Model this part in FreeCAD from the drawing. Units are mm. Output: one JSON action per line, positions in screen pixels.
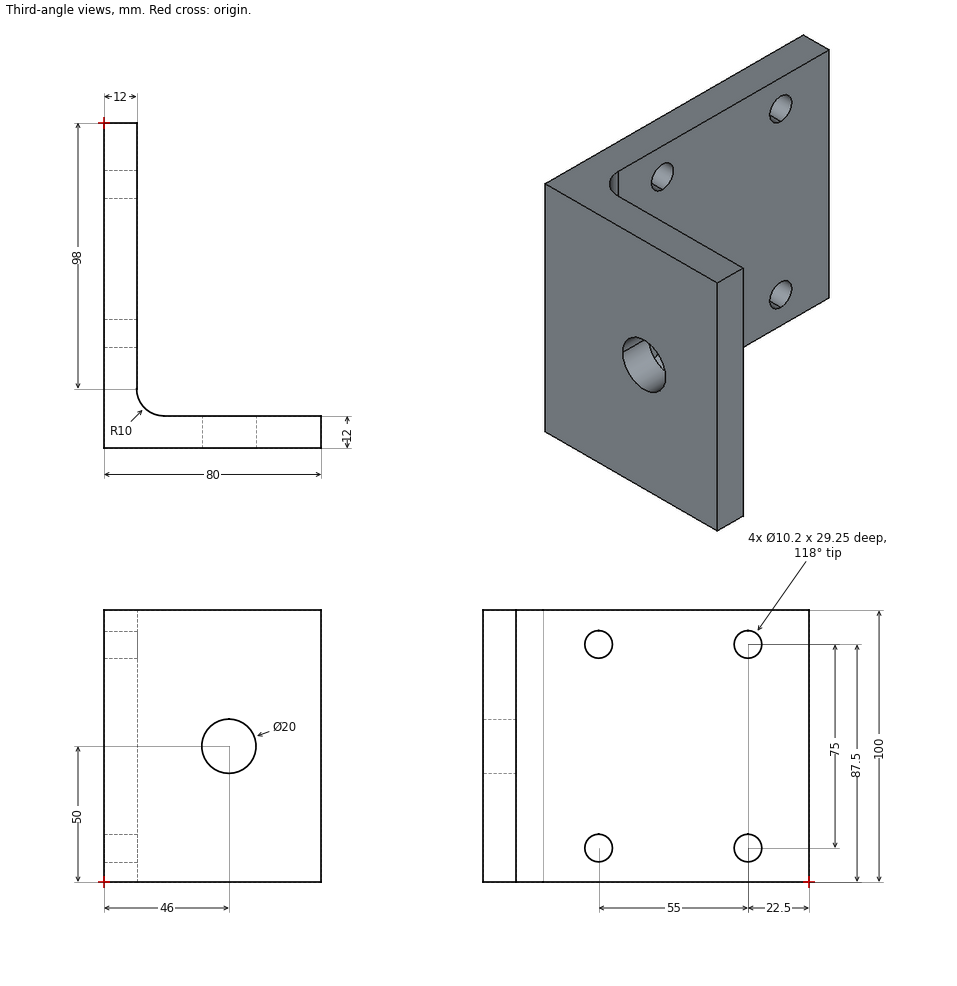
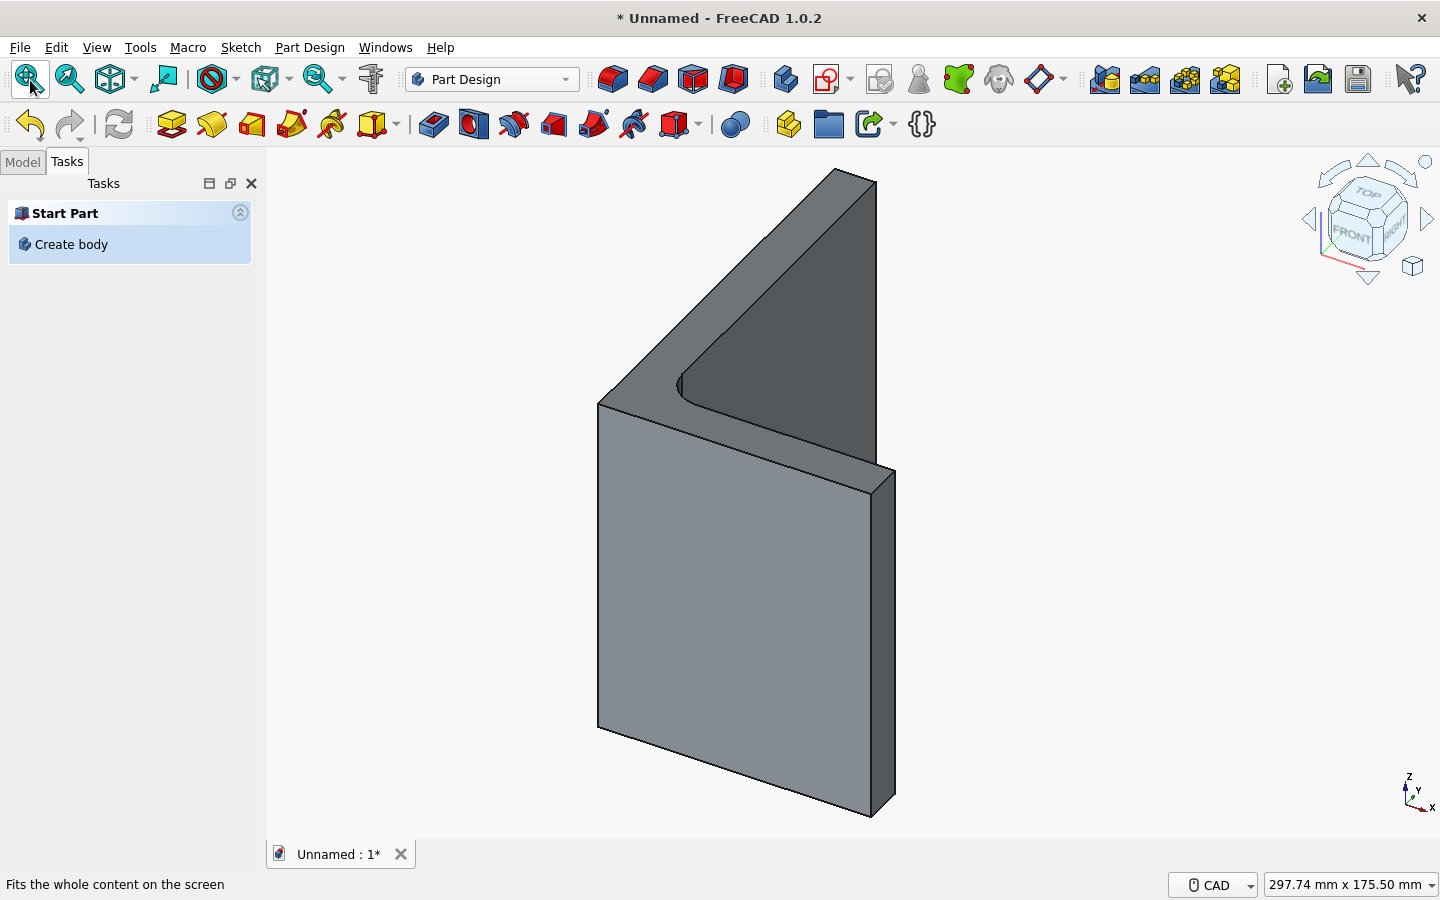
{"action": "left_click", "coordinate": [779, 393]}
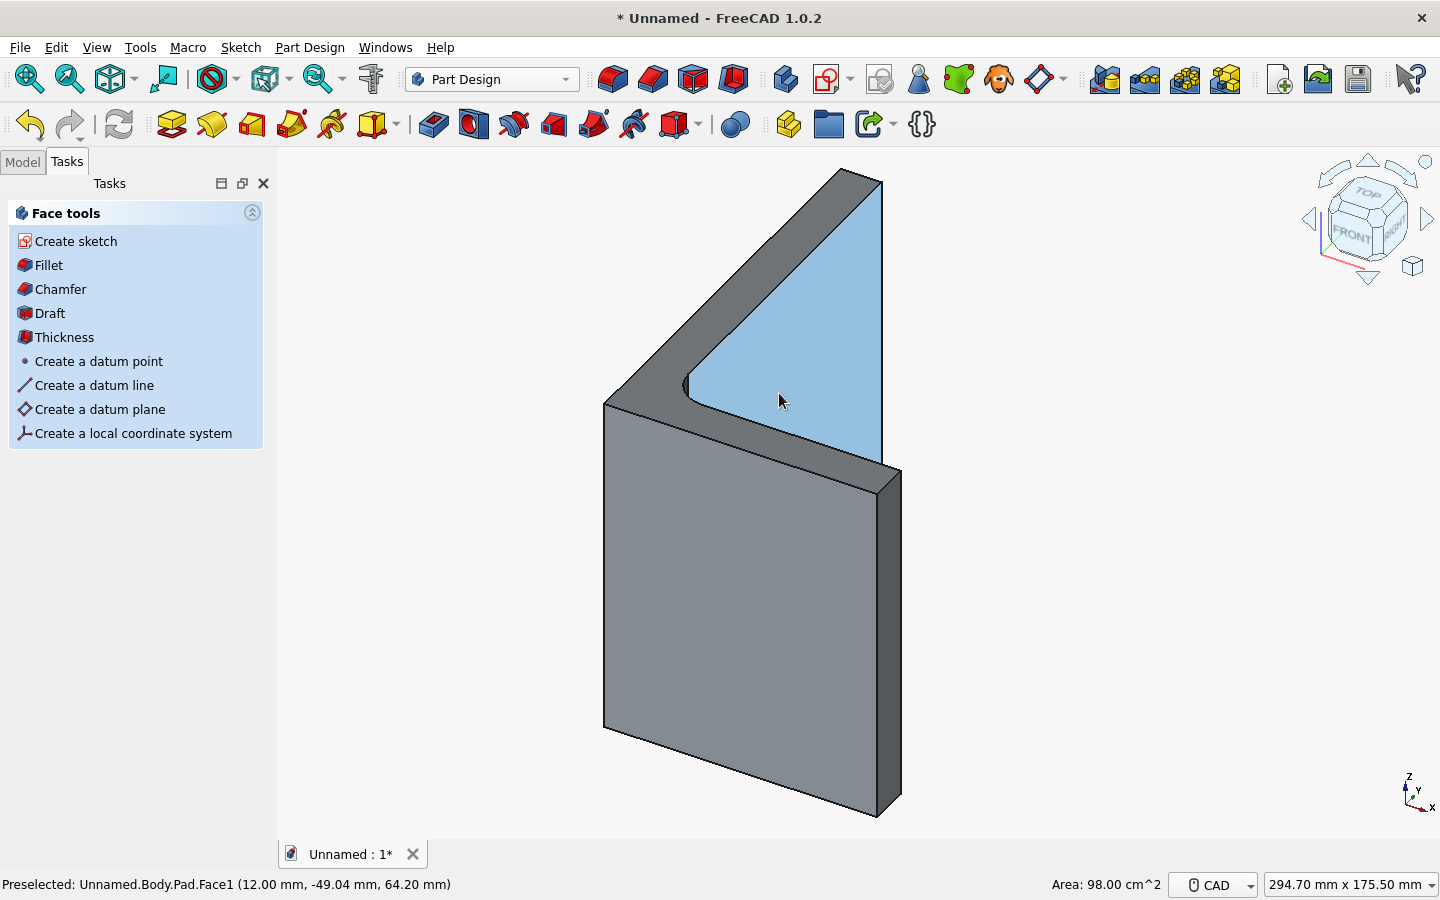
{"action": "left_click", "coordinate": [826, 80]}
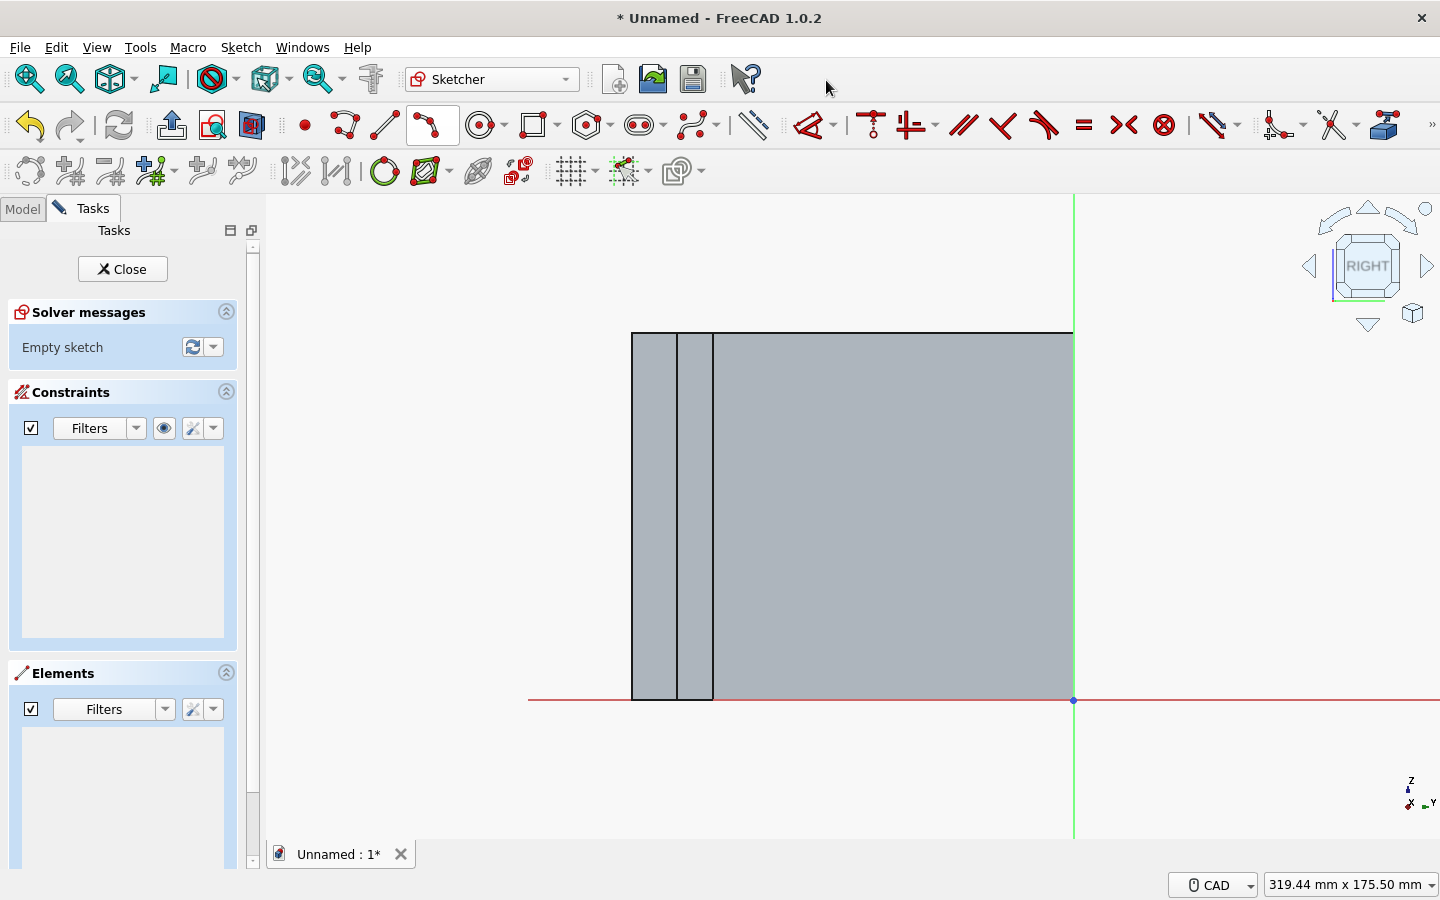
{"action": "left_click", "coordinate": [252, 126]}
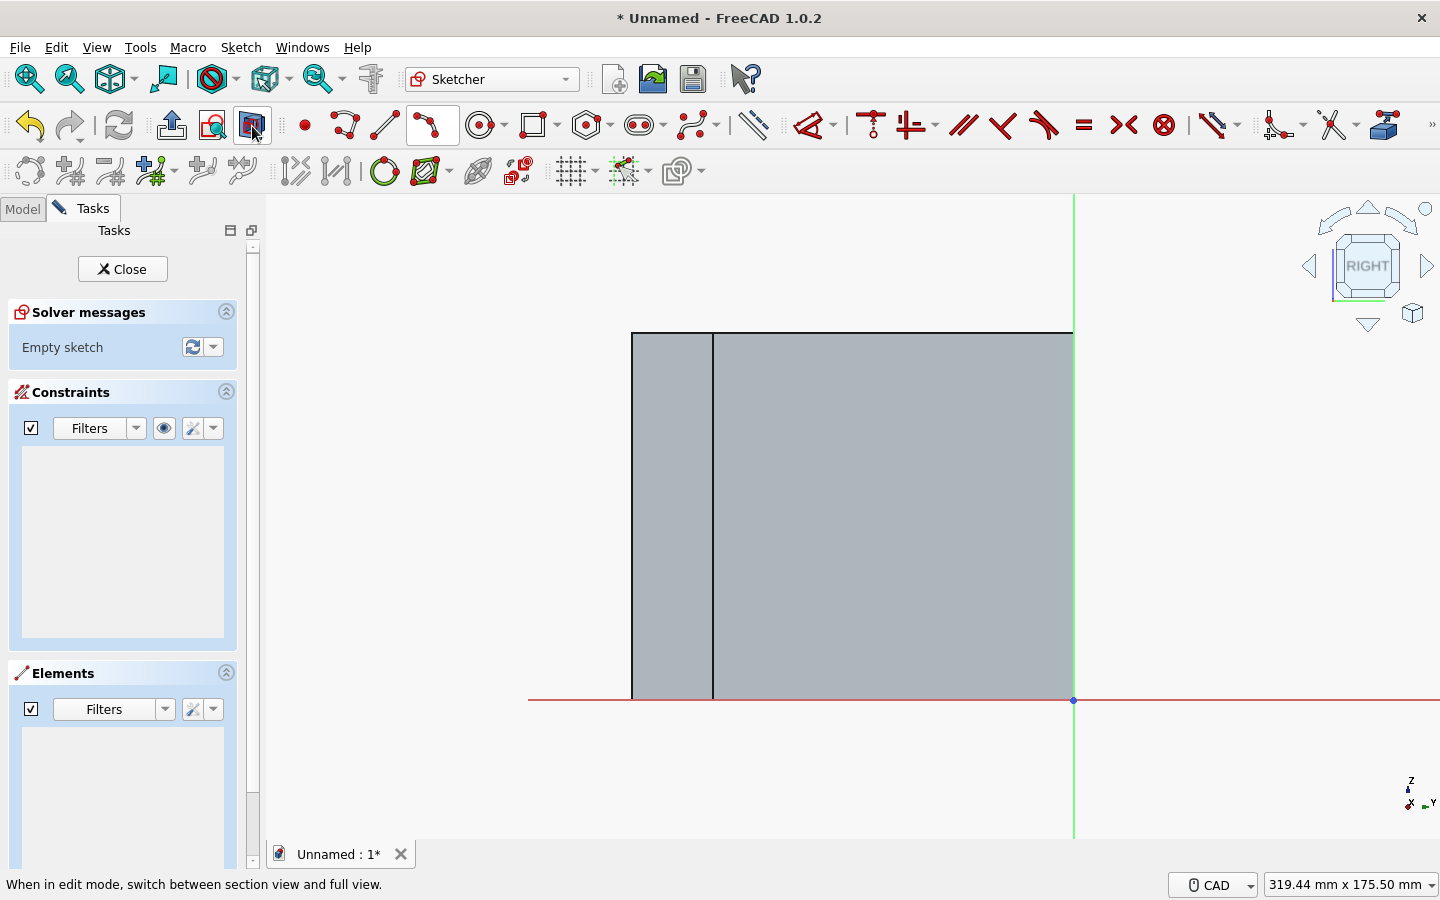
{"action": "left_click", "coordinate": [480, 126]}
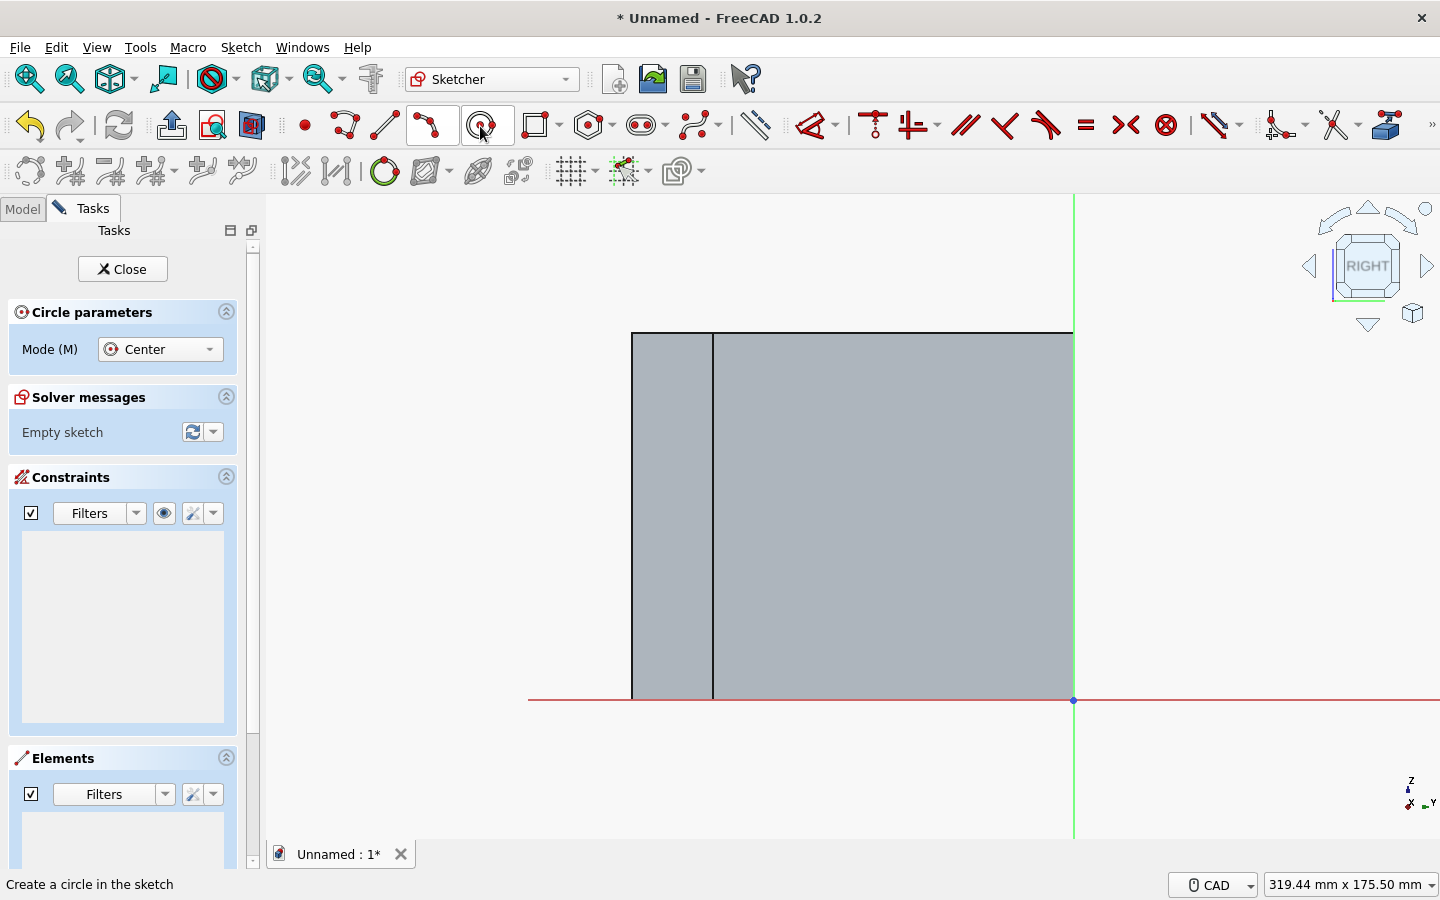
{"action": "left_click", "coordinate": [991, 379]}
{"action": "mouse_move", "coordinate": [1004, 365]}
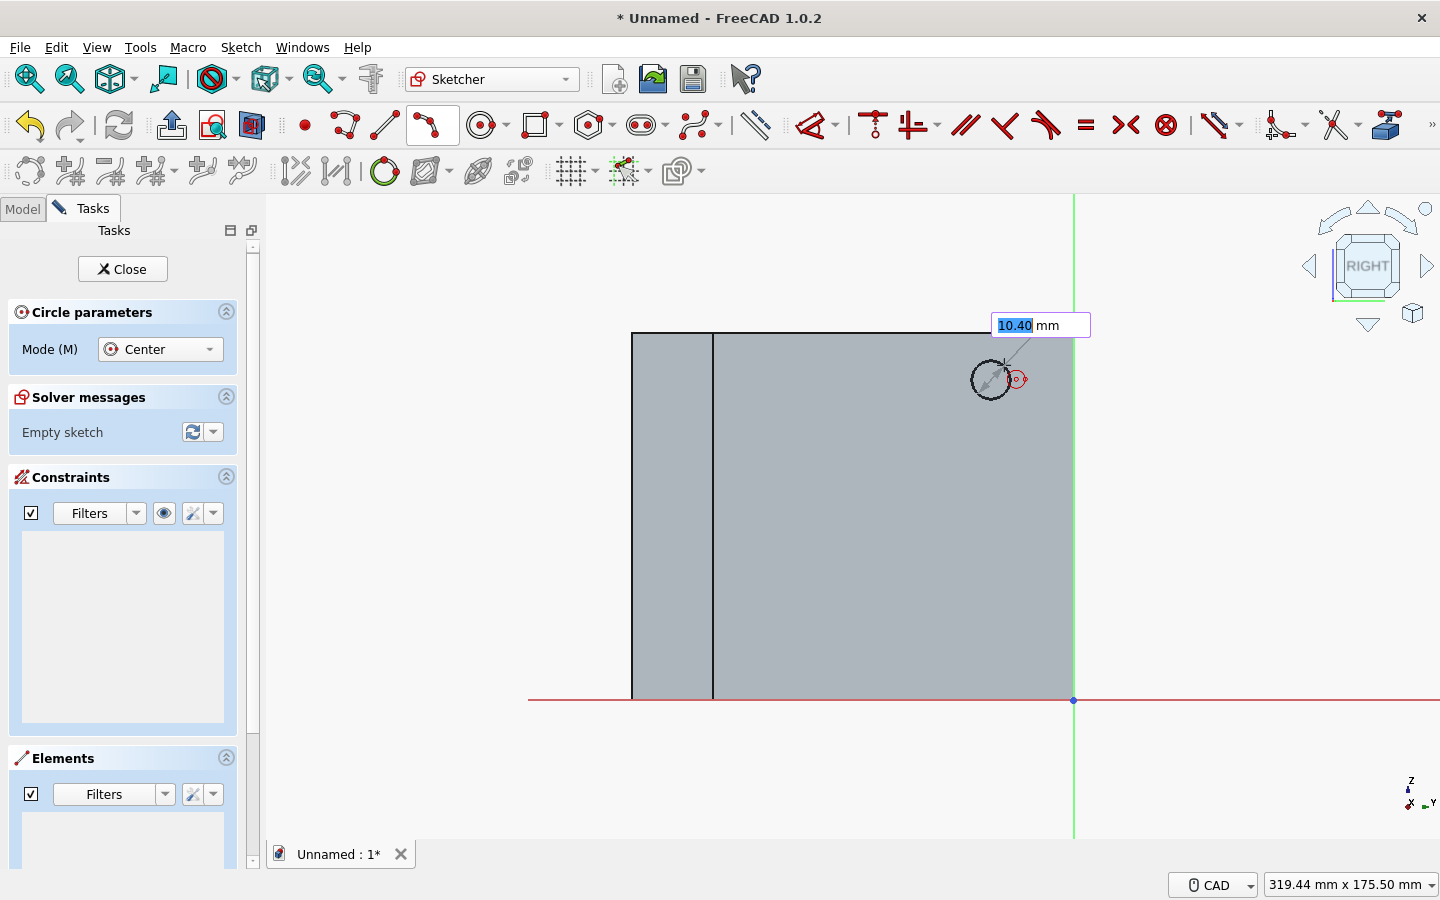
{"action": "type", "text": "10.2"}
{"action": "key", "text": "Return"}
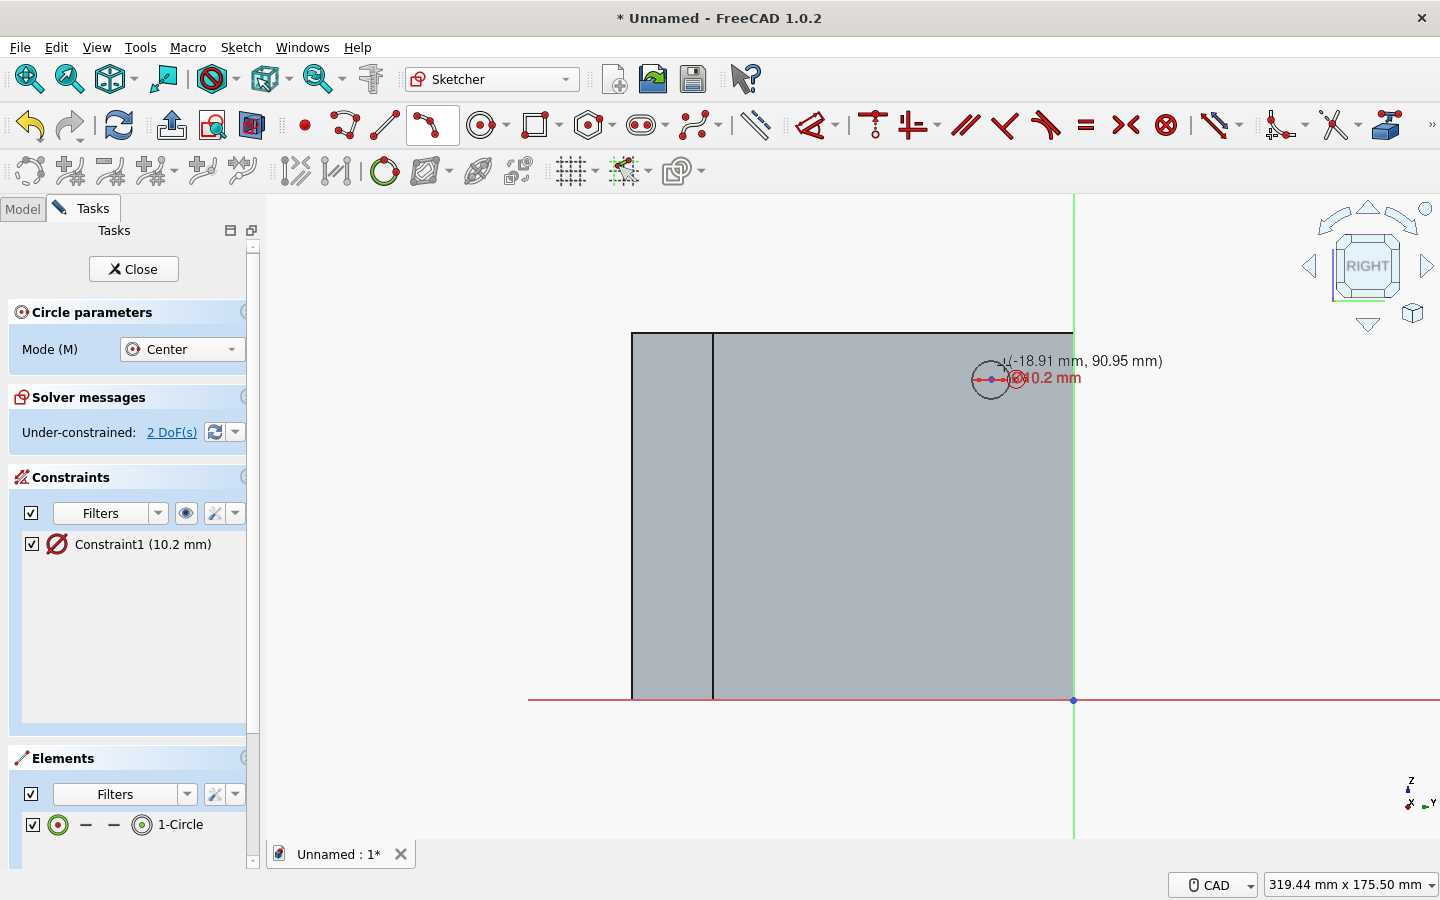
{"action": "left_click", "coordinate": [991, 654]}
{"action": "mouse_move", "coordinate": [1004, 641]}